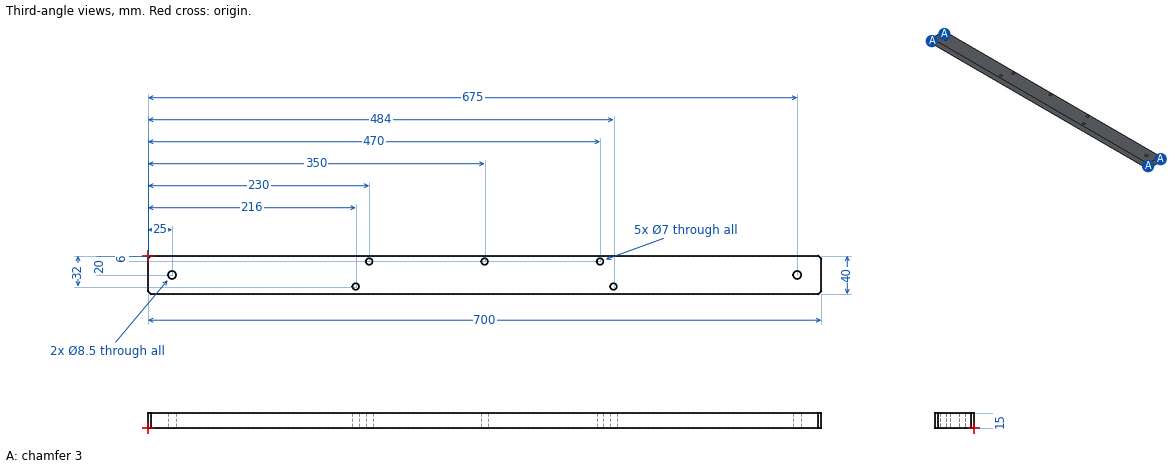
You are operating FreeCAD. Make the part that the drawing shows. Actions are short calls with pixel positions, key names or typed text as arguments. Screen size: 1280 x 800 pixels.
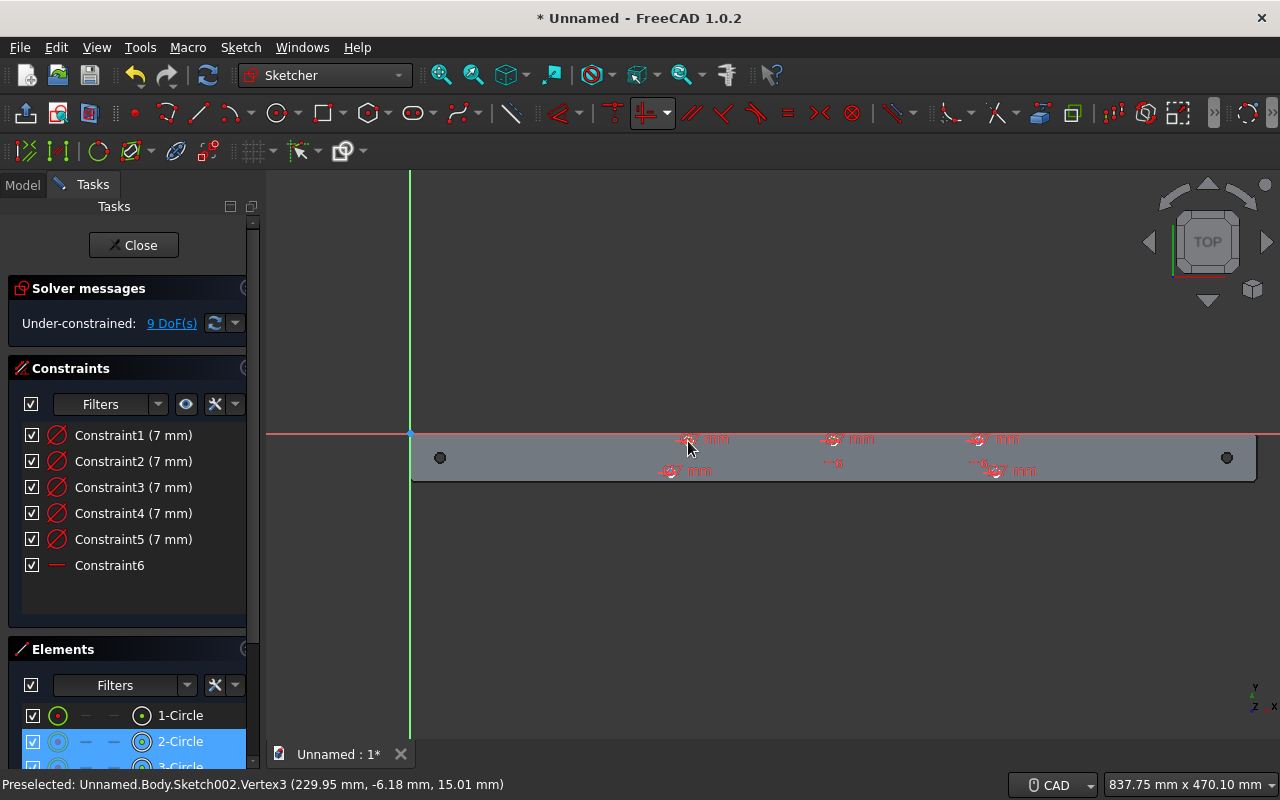
click(670, 114)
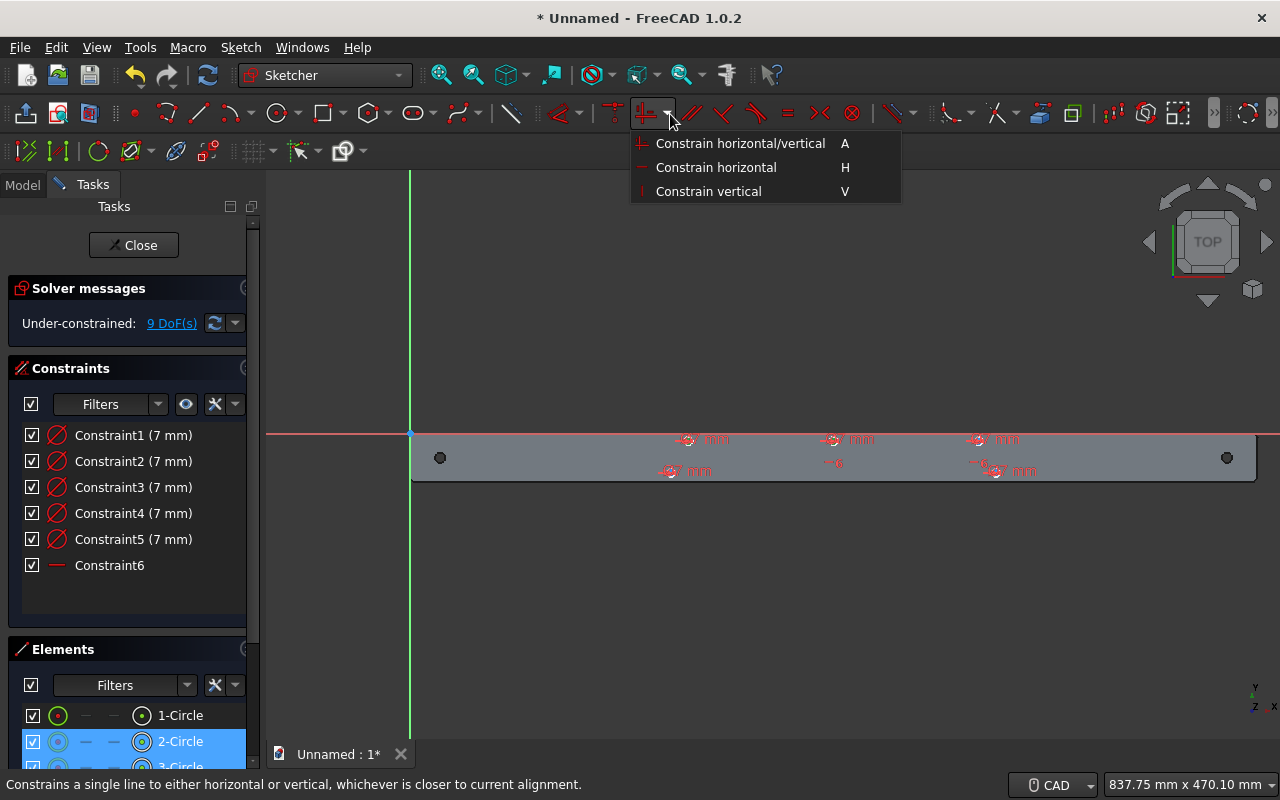
click(766, 167)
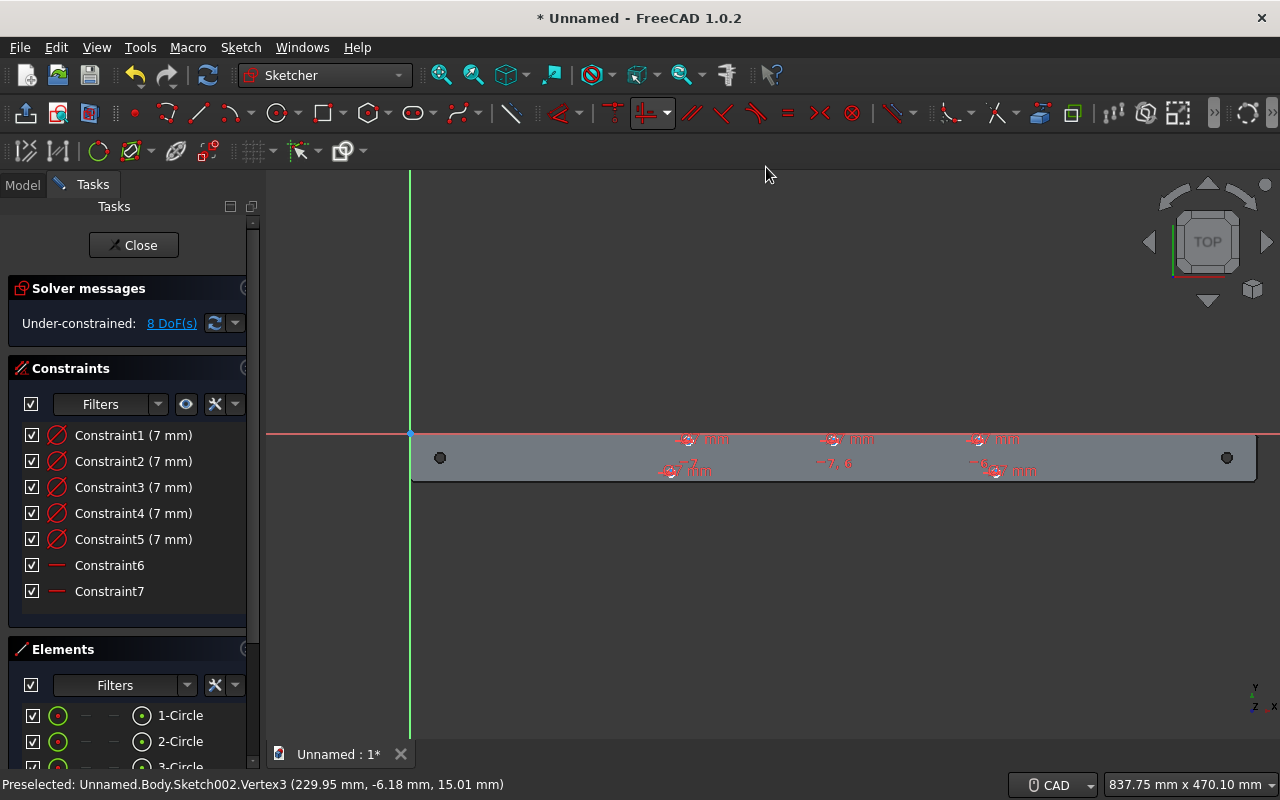
click(671, 473)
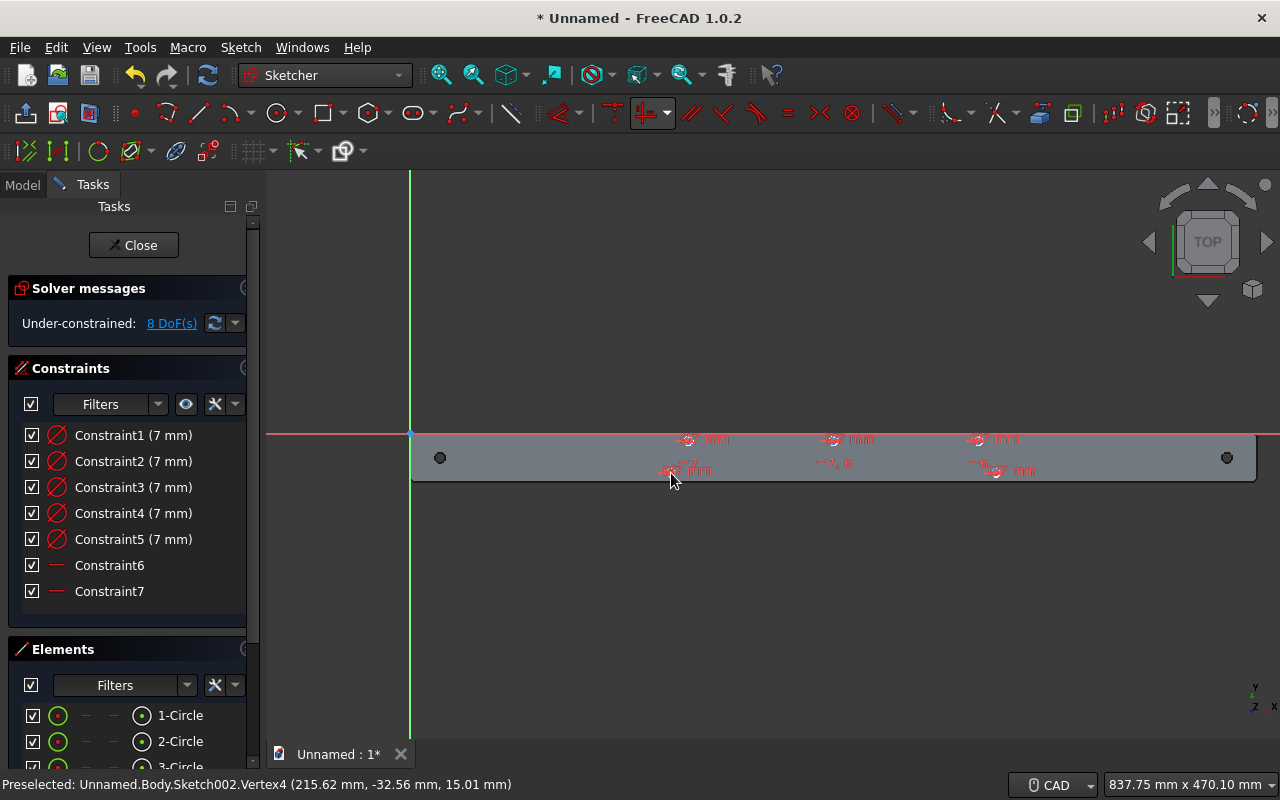
click(996, 473)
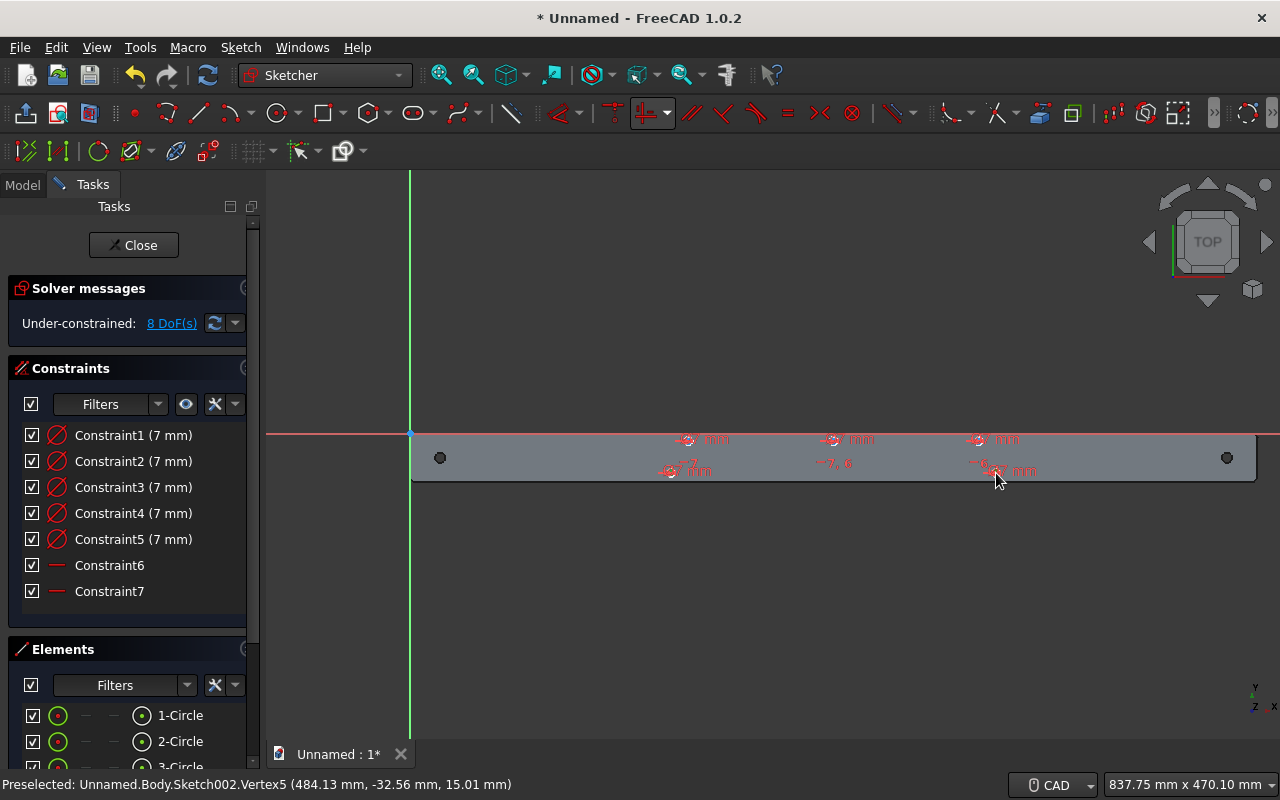
key(h)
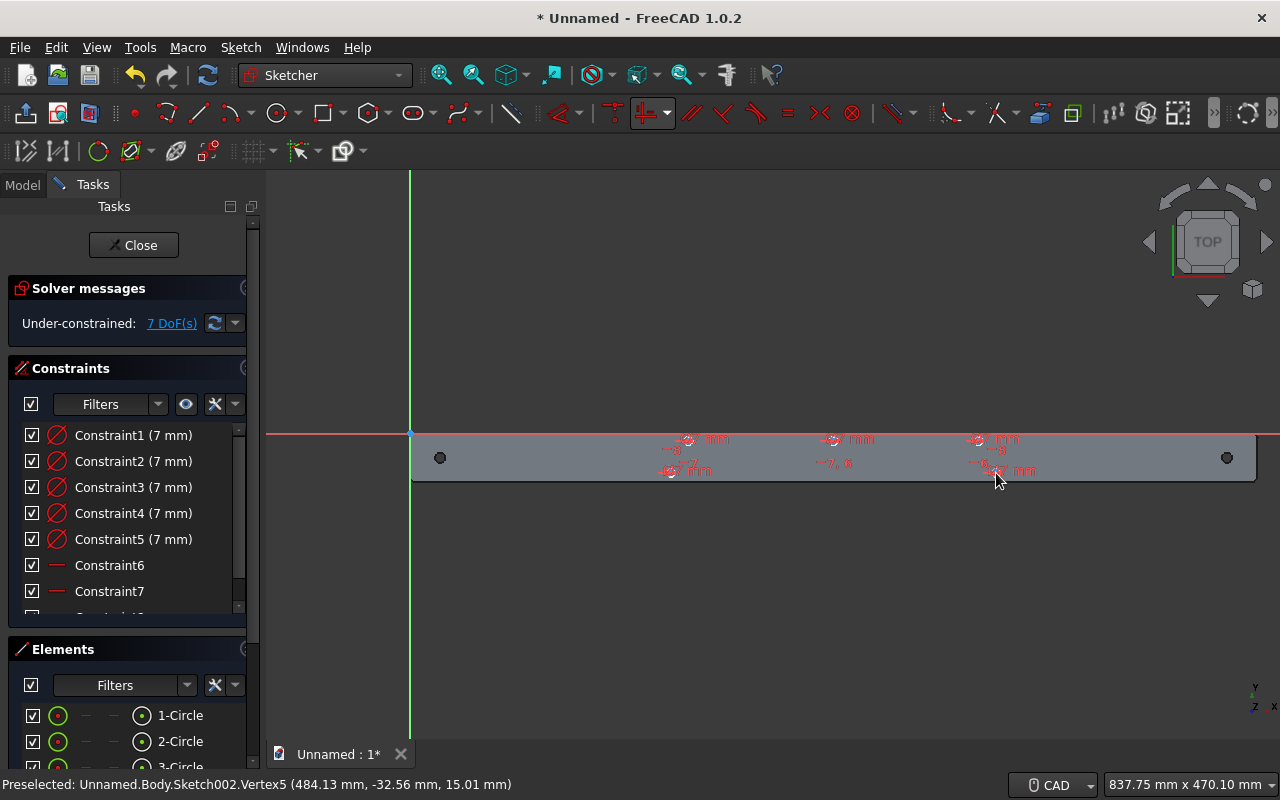
click(558, 114)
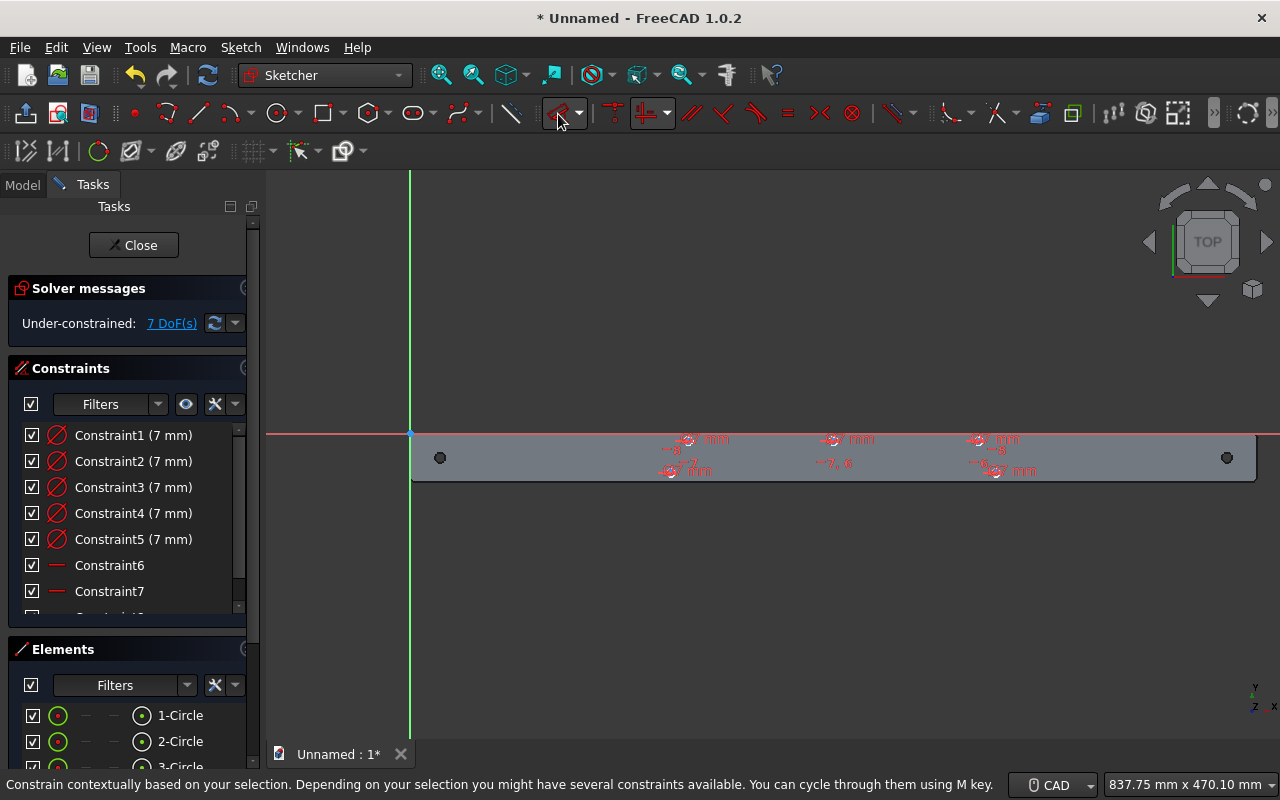
scroll(979, 441, up, 9)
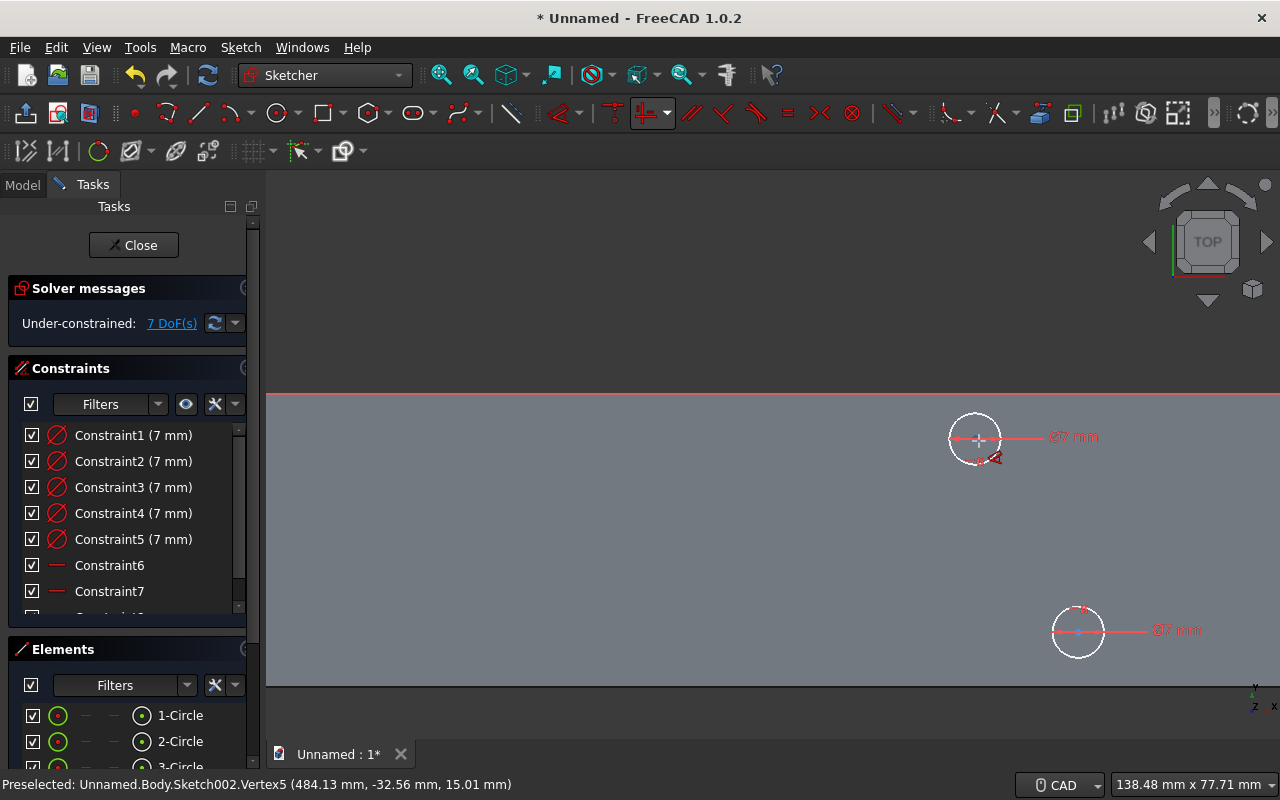
click(975, 439)
click(1009, 416)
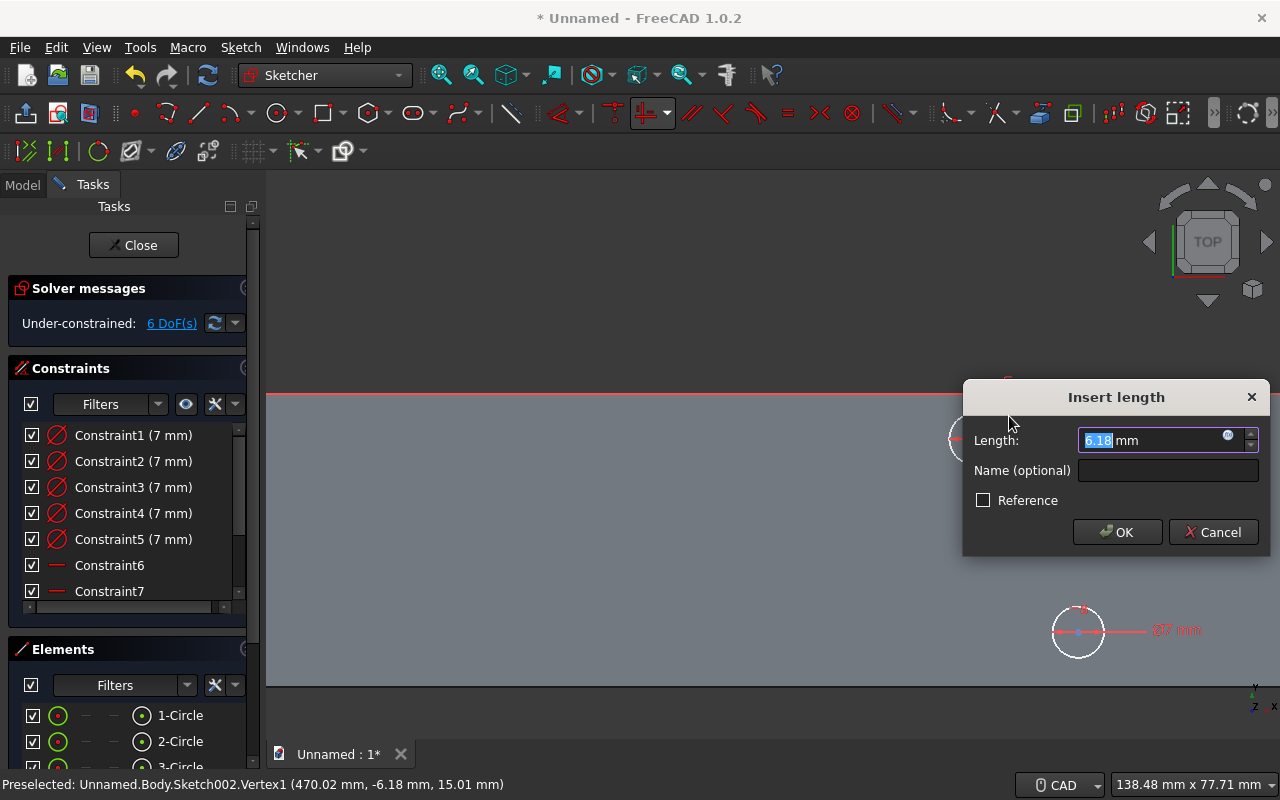
text(6)
key(Return)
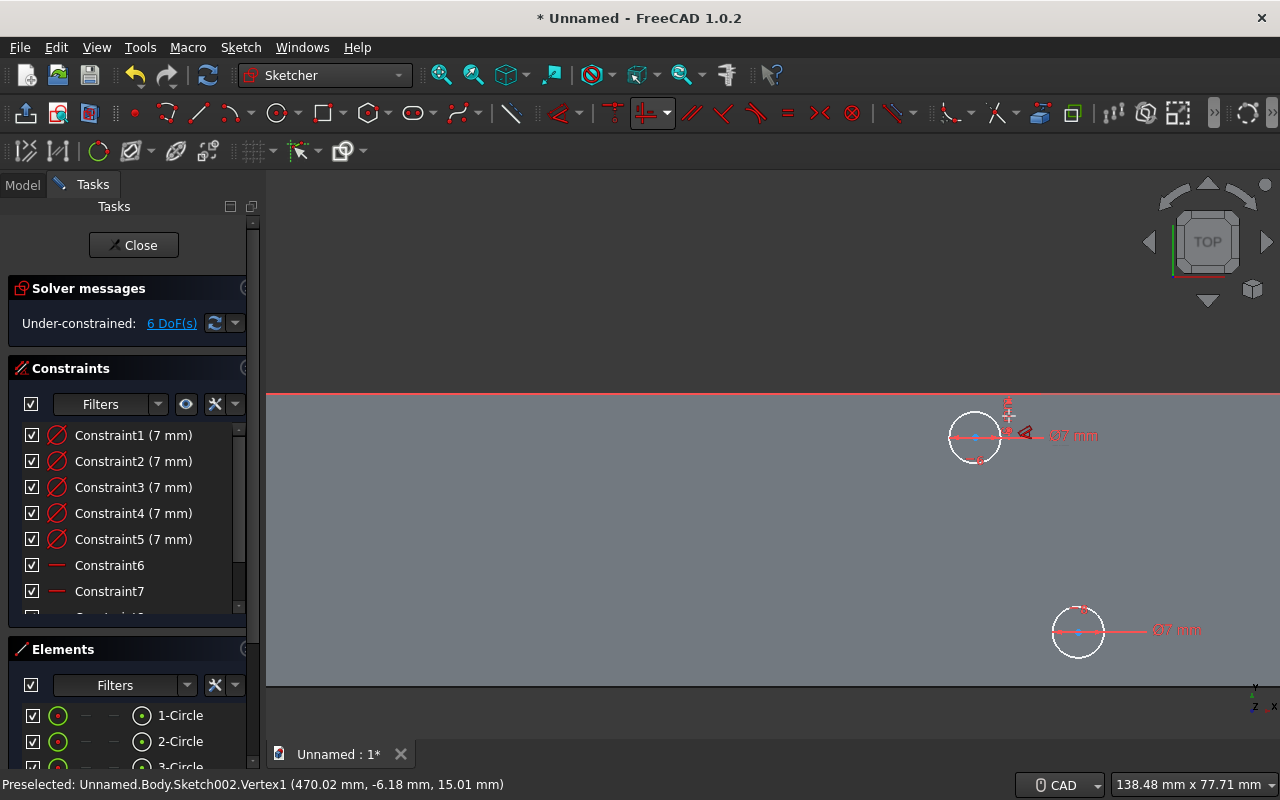
scroll(979, 441, down, 9)